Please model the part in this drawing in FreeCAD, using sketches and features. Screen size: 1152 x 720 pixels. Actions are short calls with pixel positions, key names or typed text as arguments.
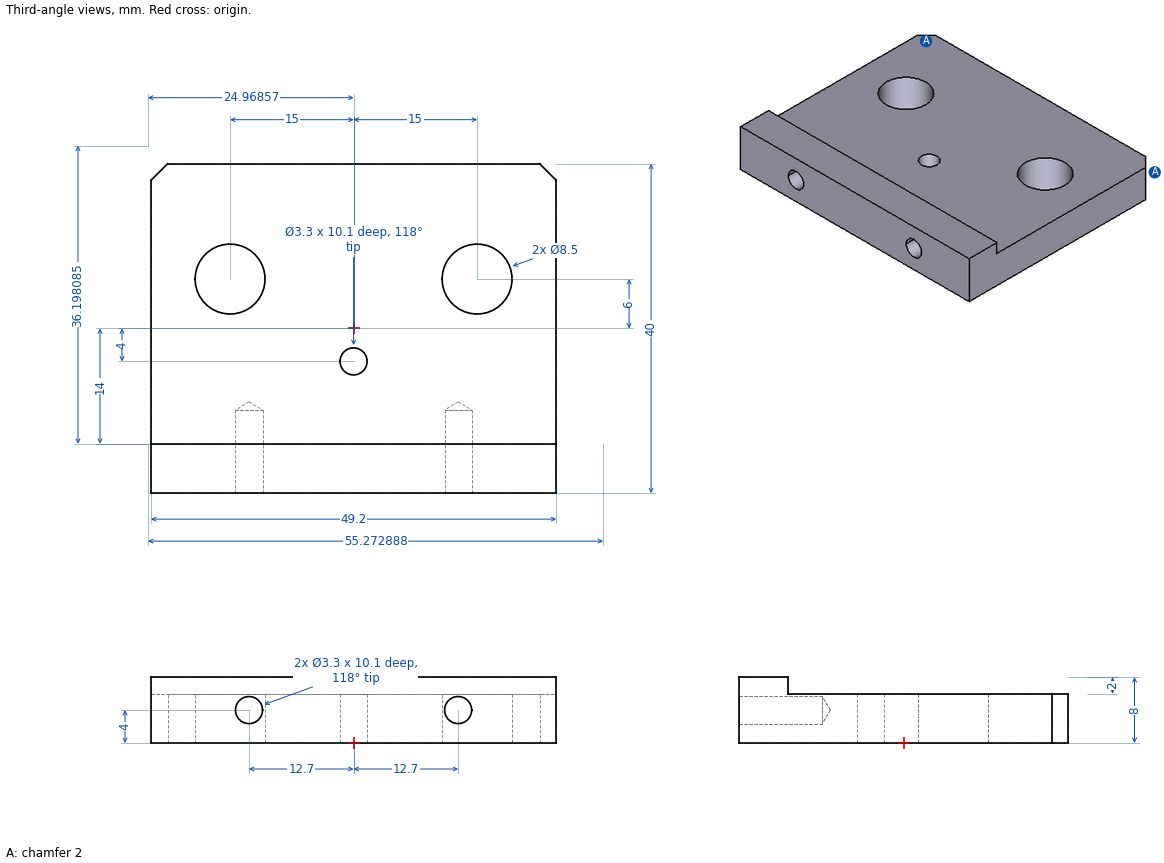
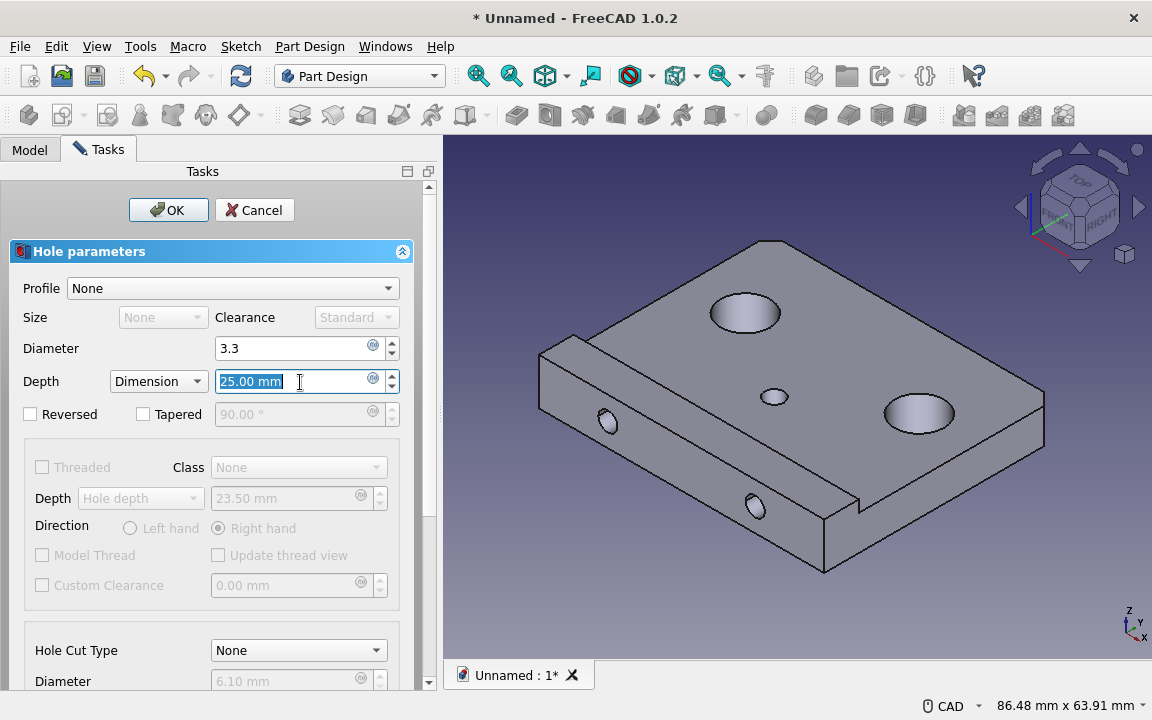
text(10.1)
key(Tab)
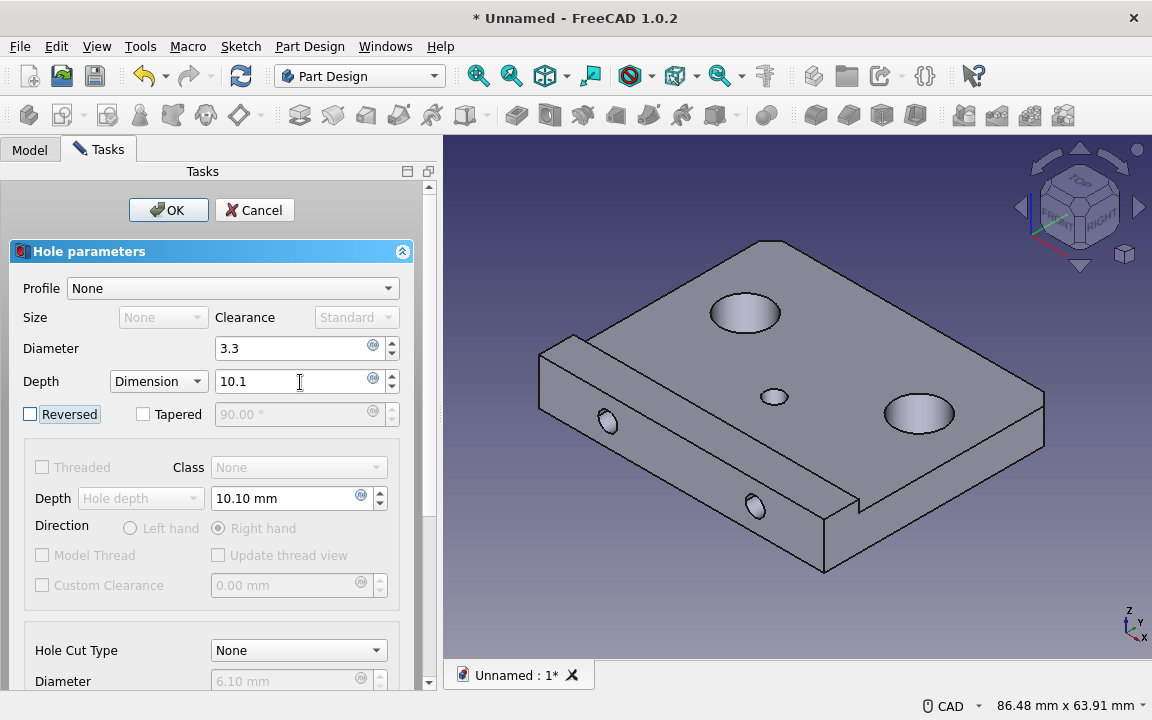
click(169, 210)